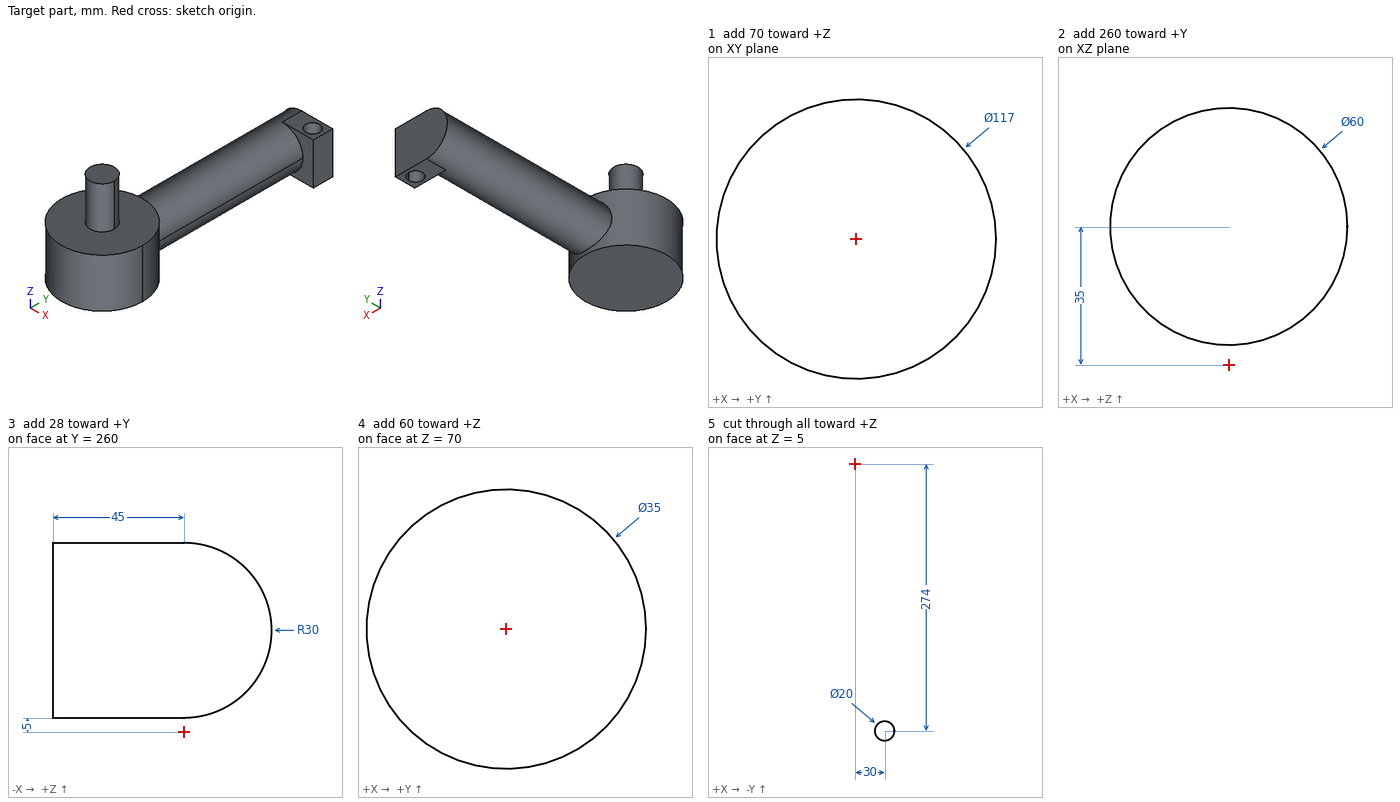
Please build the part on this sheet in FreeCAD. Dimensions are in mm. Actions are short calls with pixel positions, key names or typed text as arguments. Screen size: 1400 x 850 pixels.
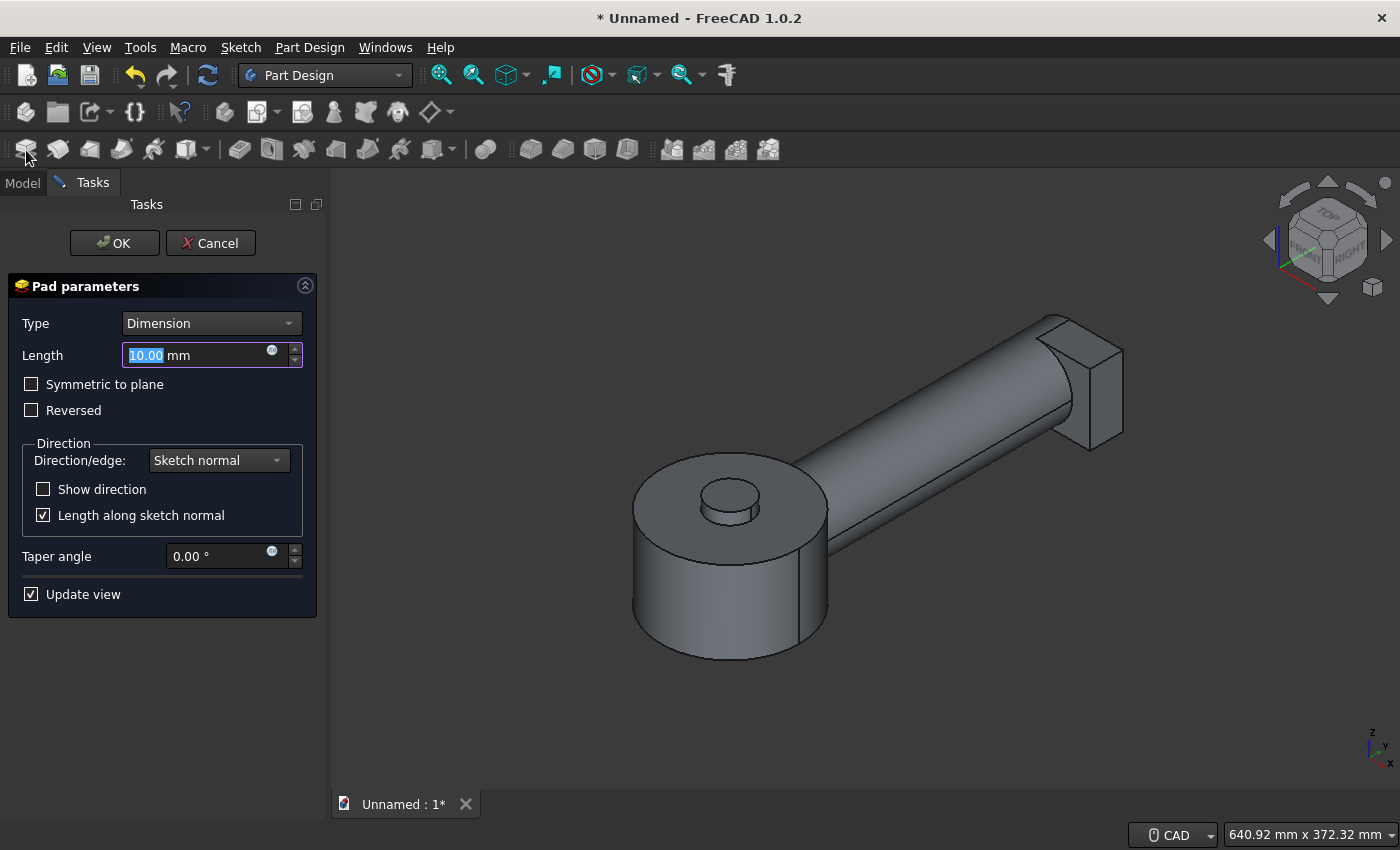
text(60)
key(Tab)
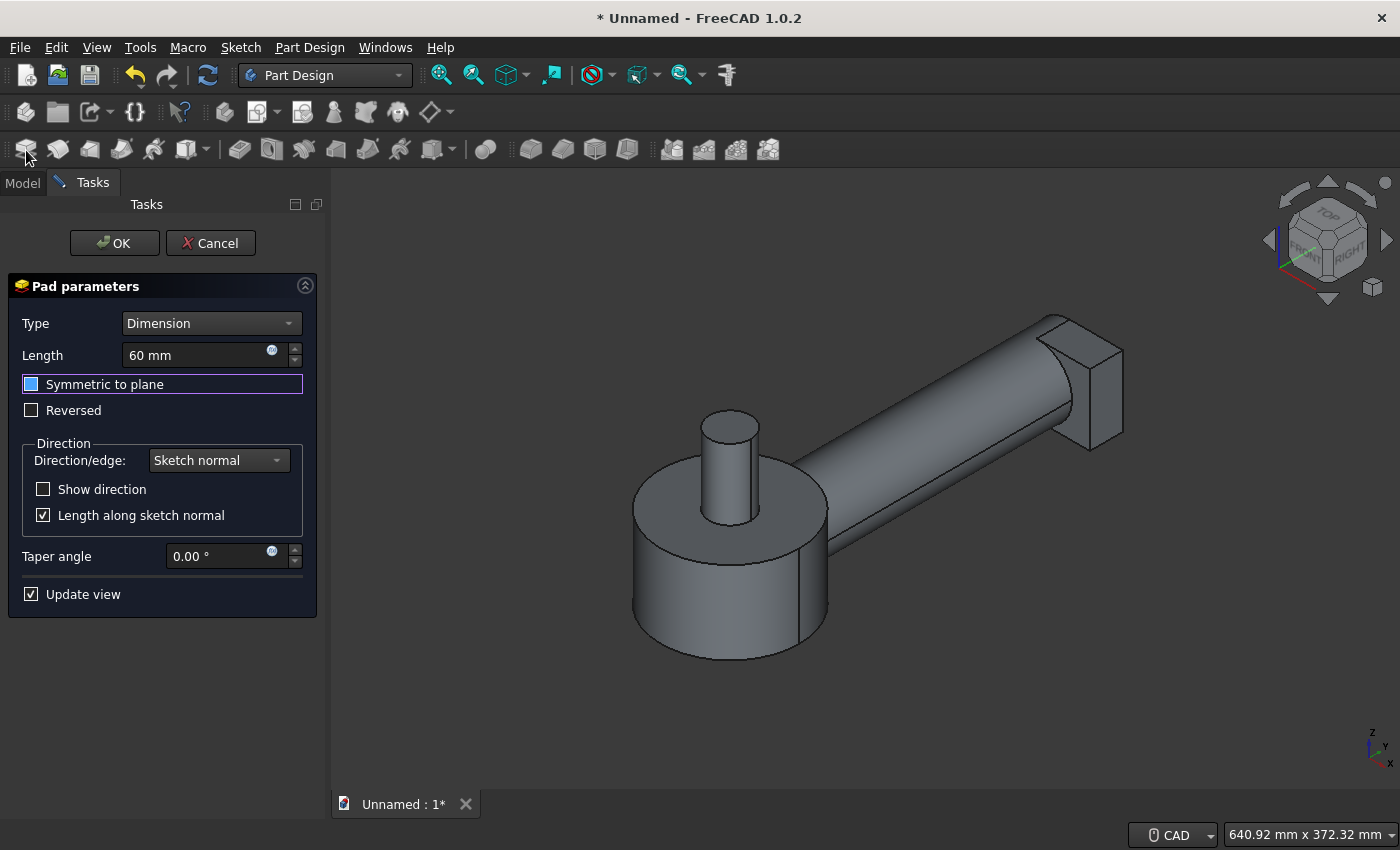
click(115, 243)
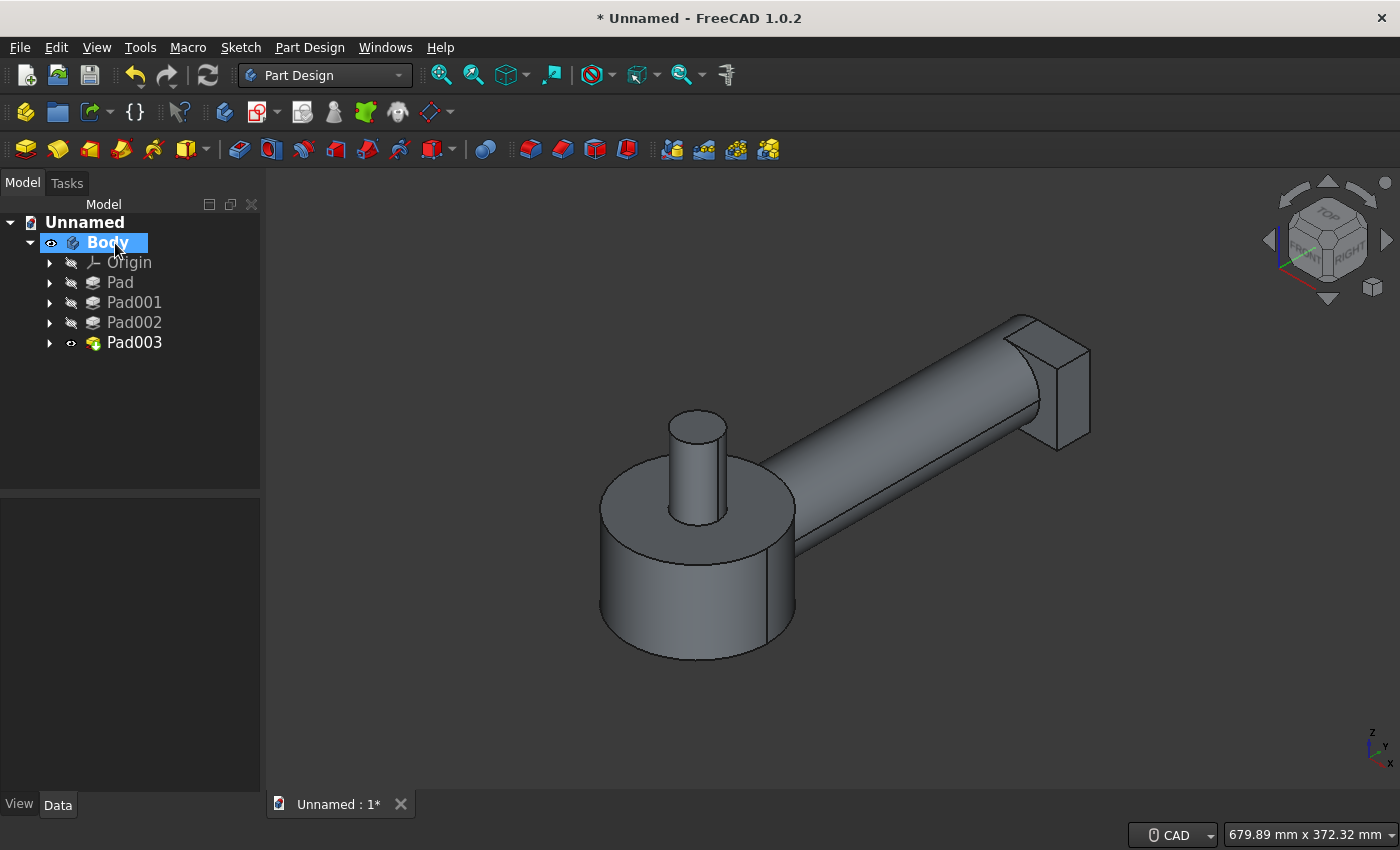
key(5)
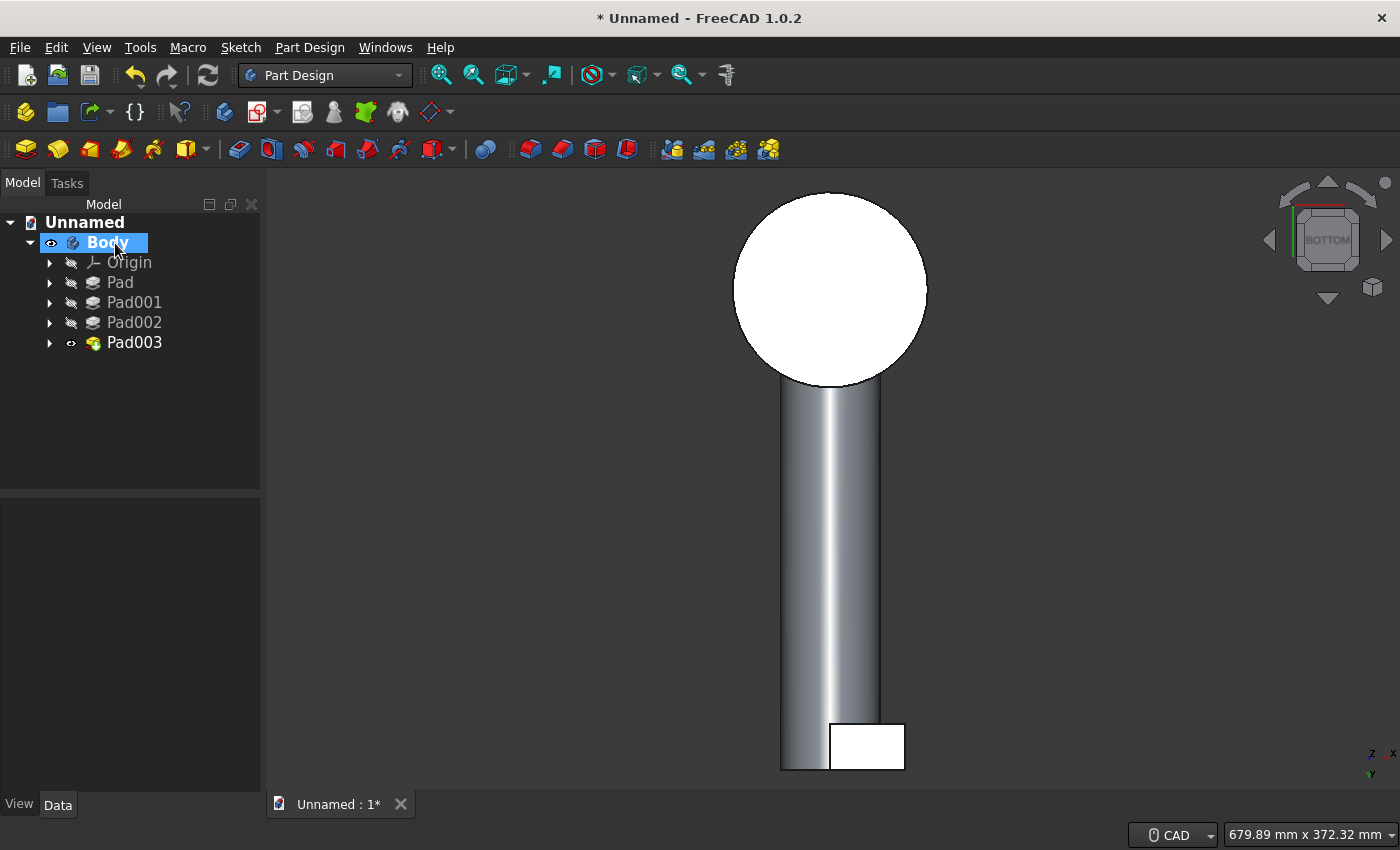
click(878, 746)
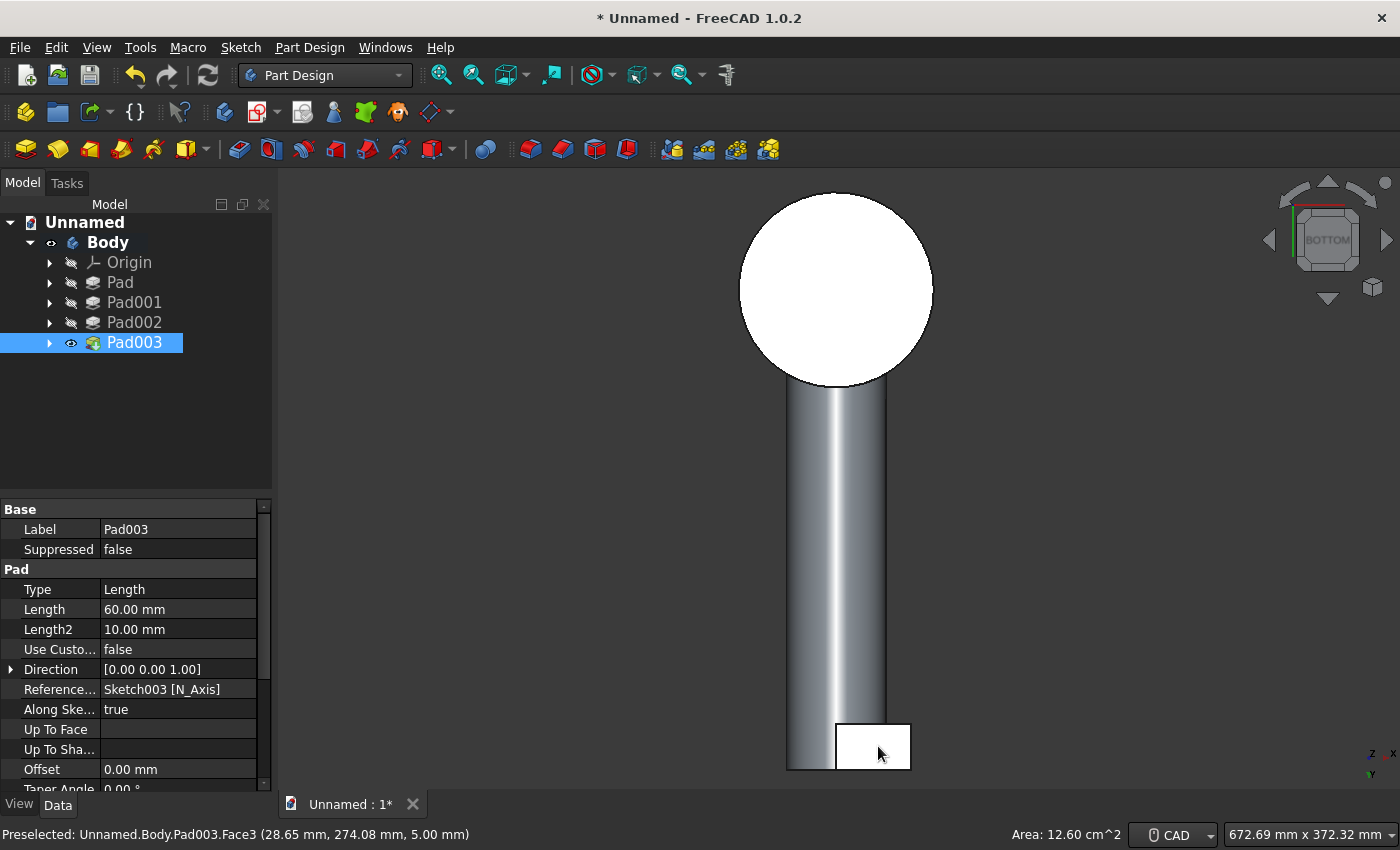
click(258, 112)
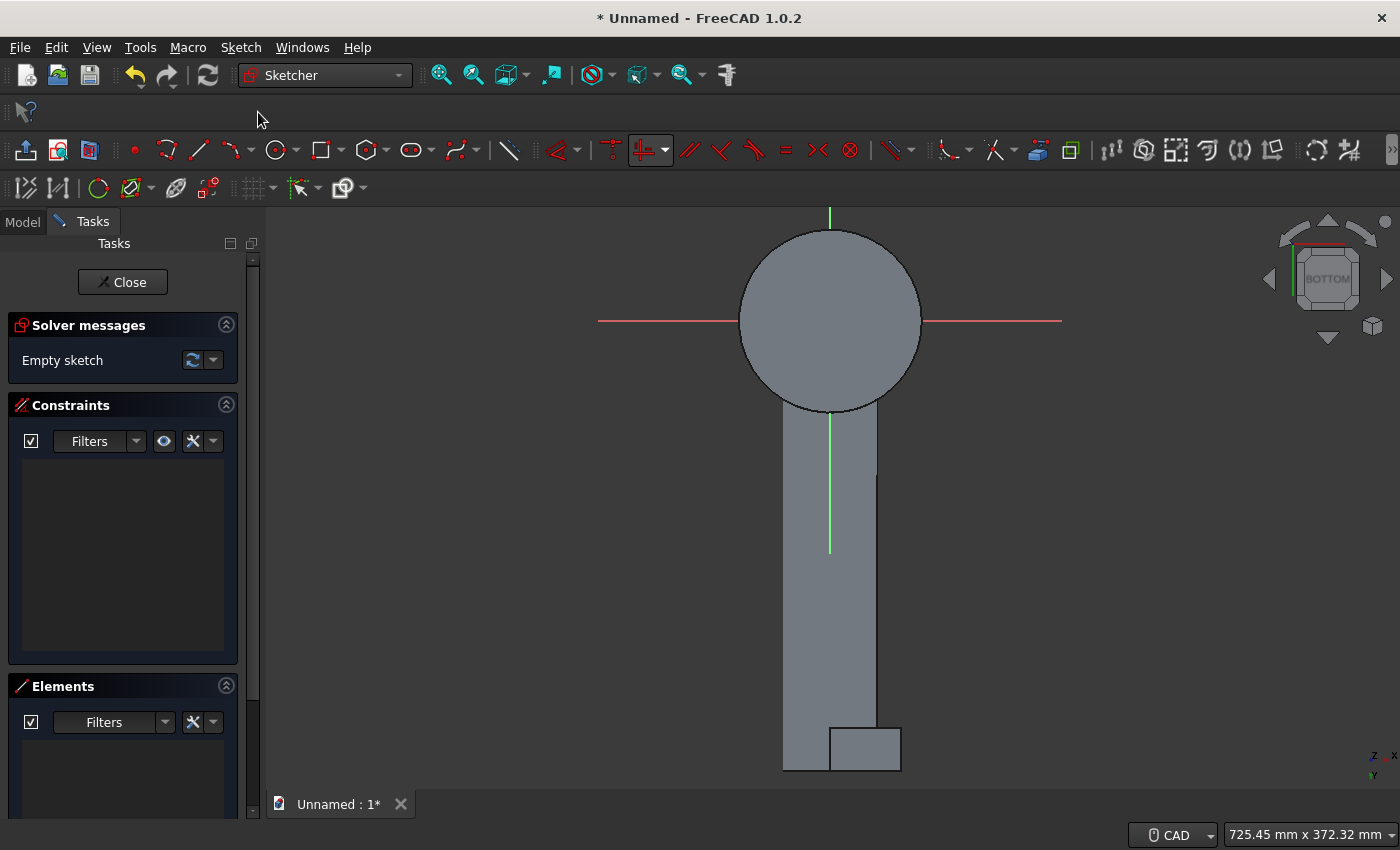
click(90, 150)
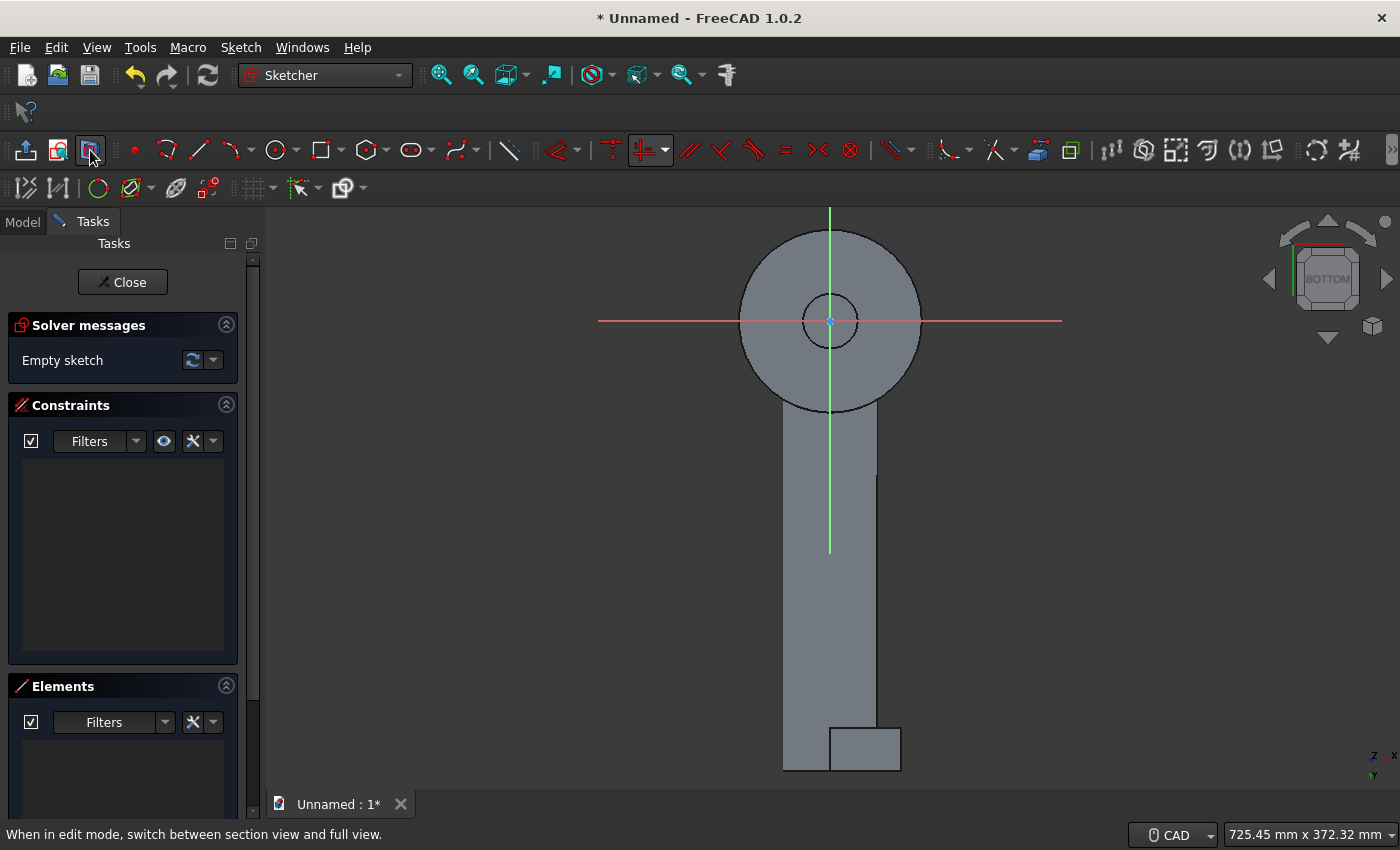
scroll(764, 498, down, 5)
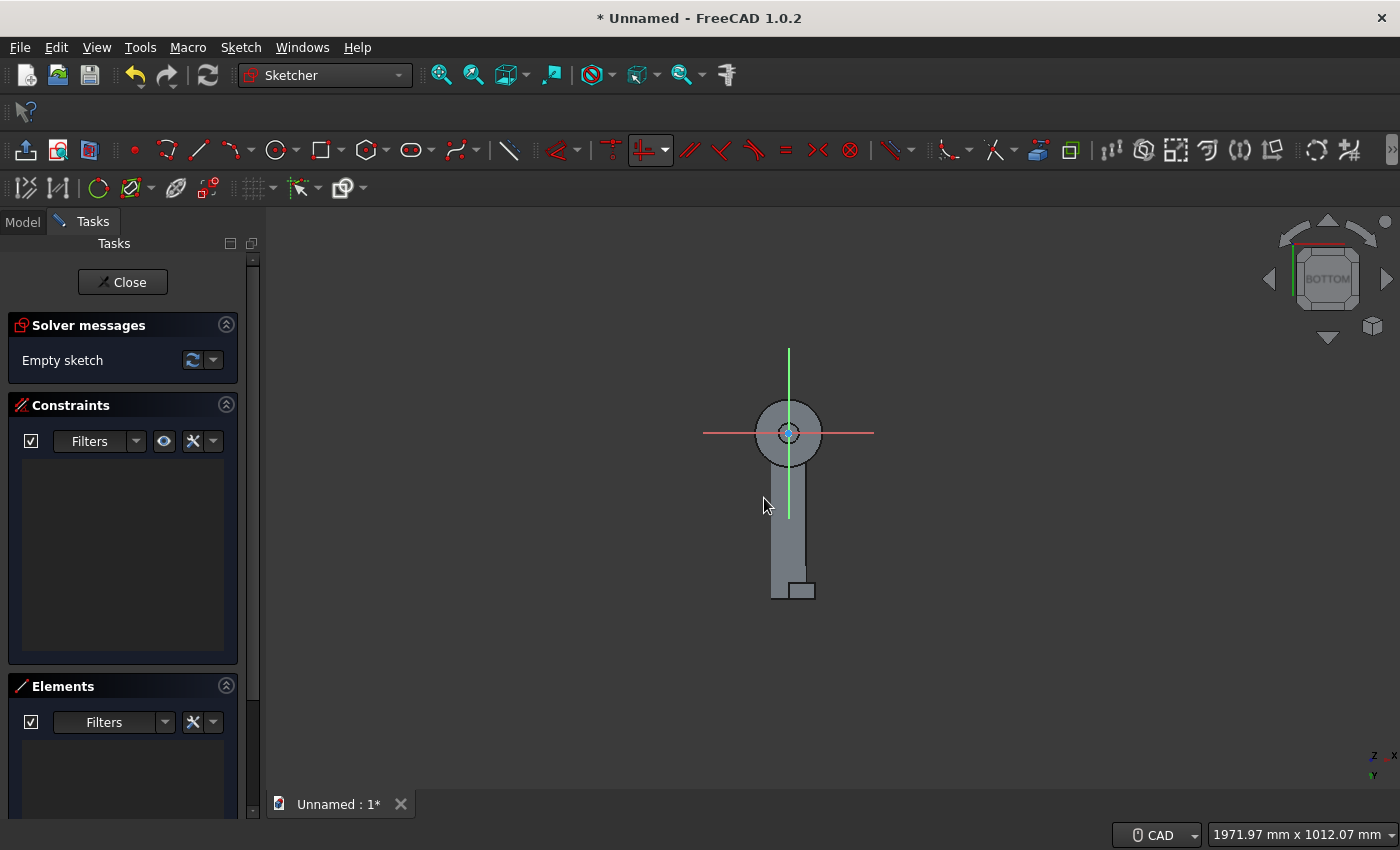
scroll(808, 596, up, 15)